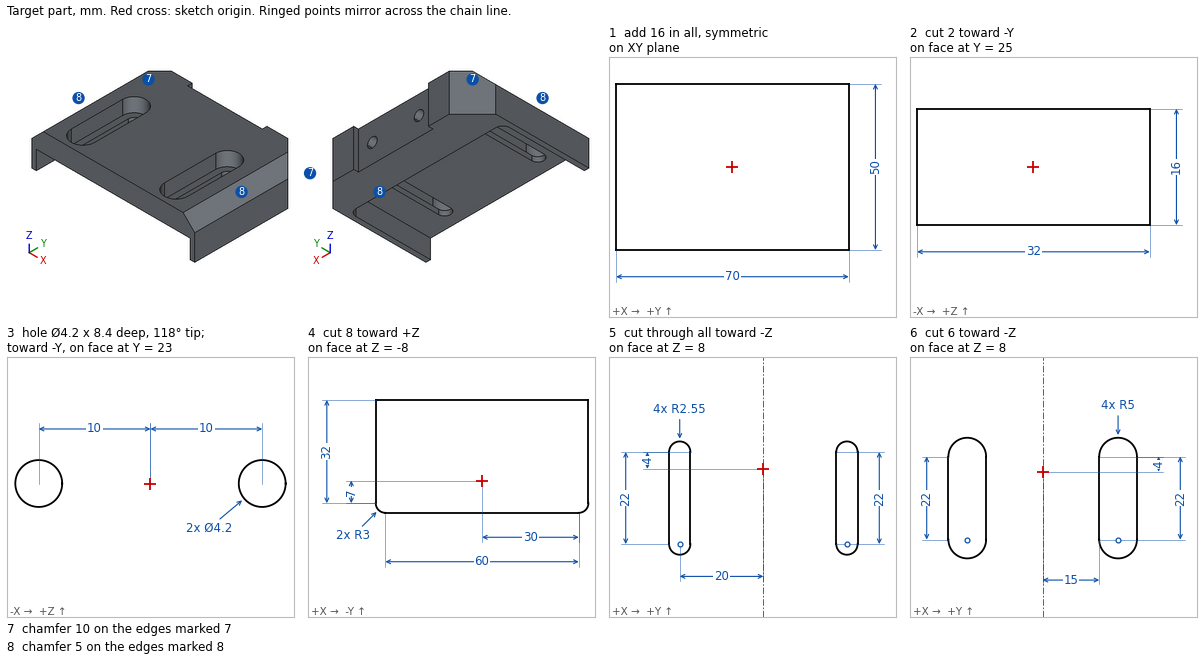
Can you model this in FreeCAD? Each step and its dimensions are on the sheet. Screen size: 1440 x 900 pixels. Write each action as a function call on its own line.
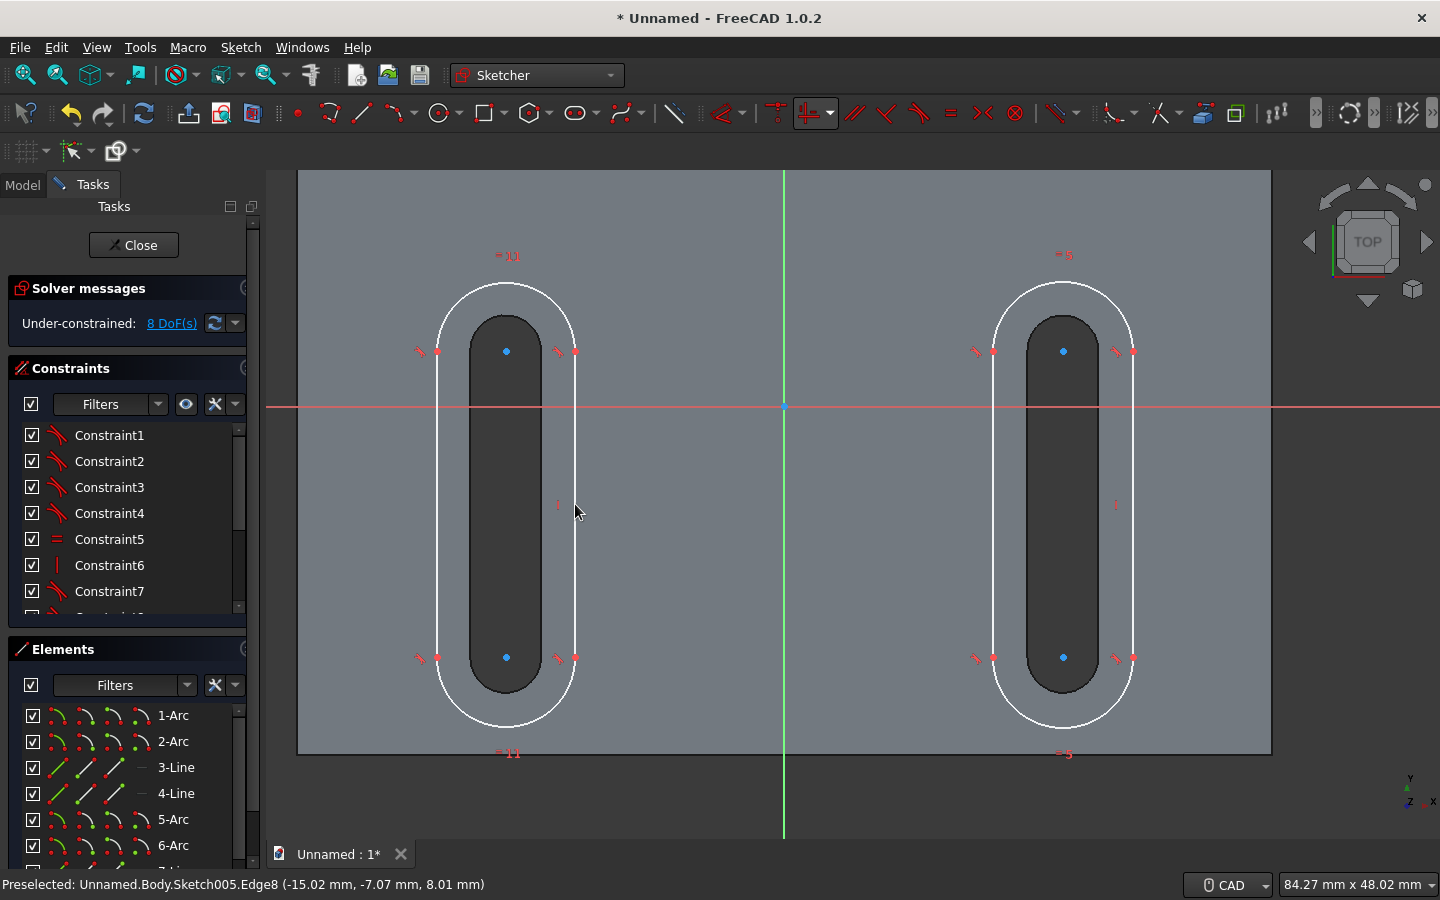
click(1022, 715)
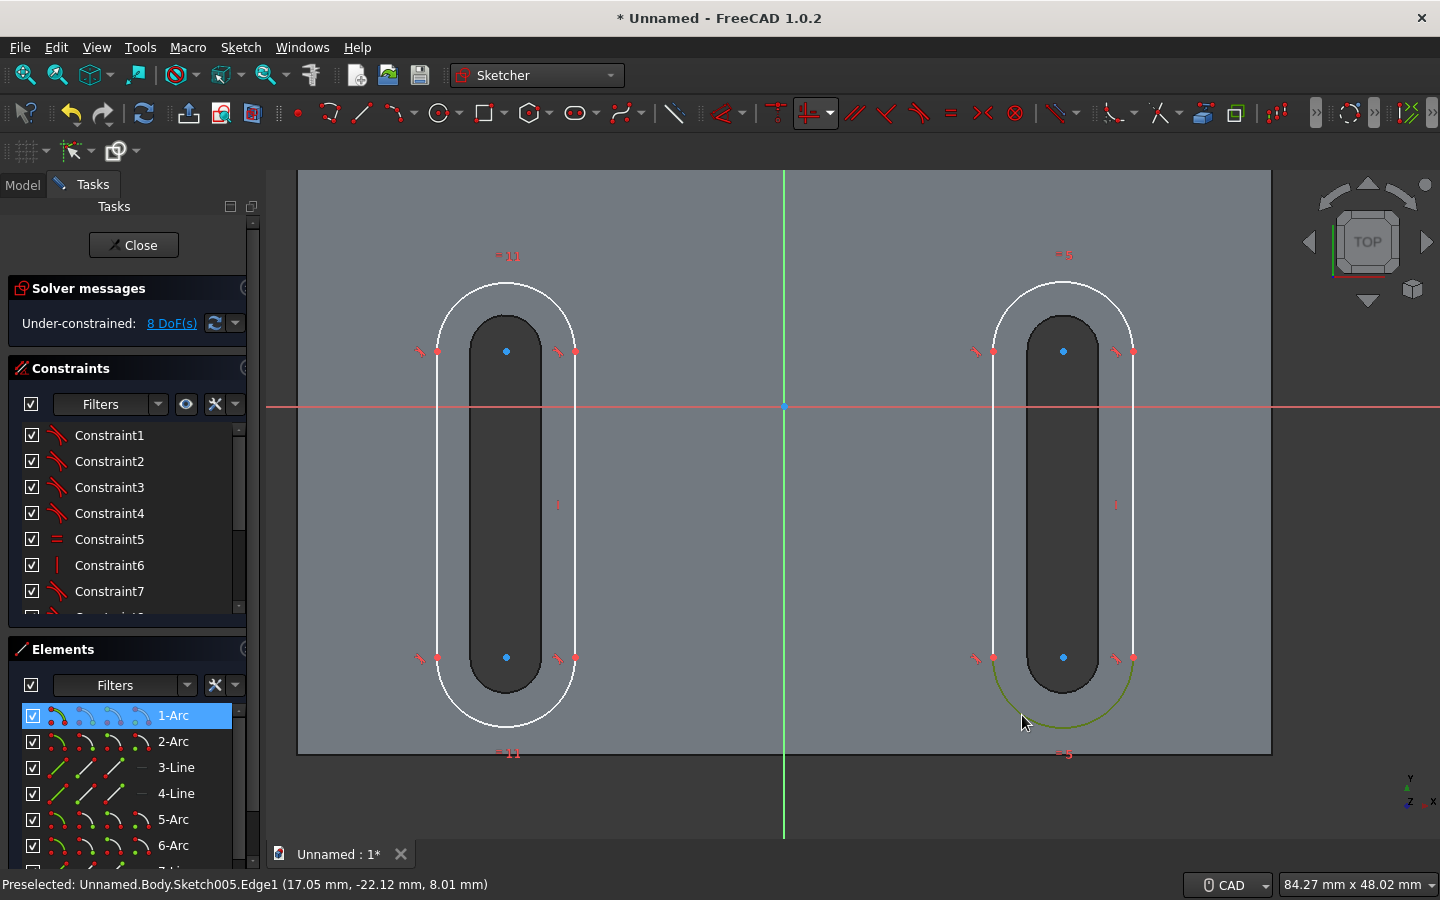
click(465, 714)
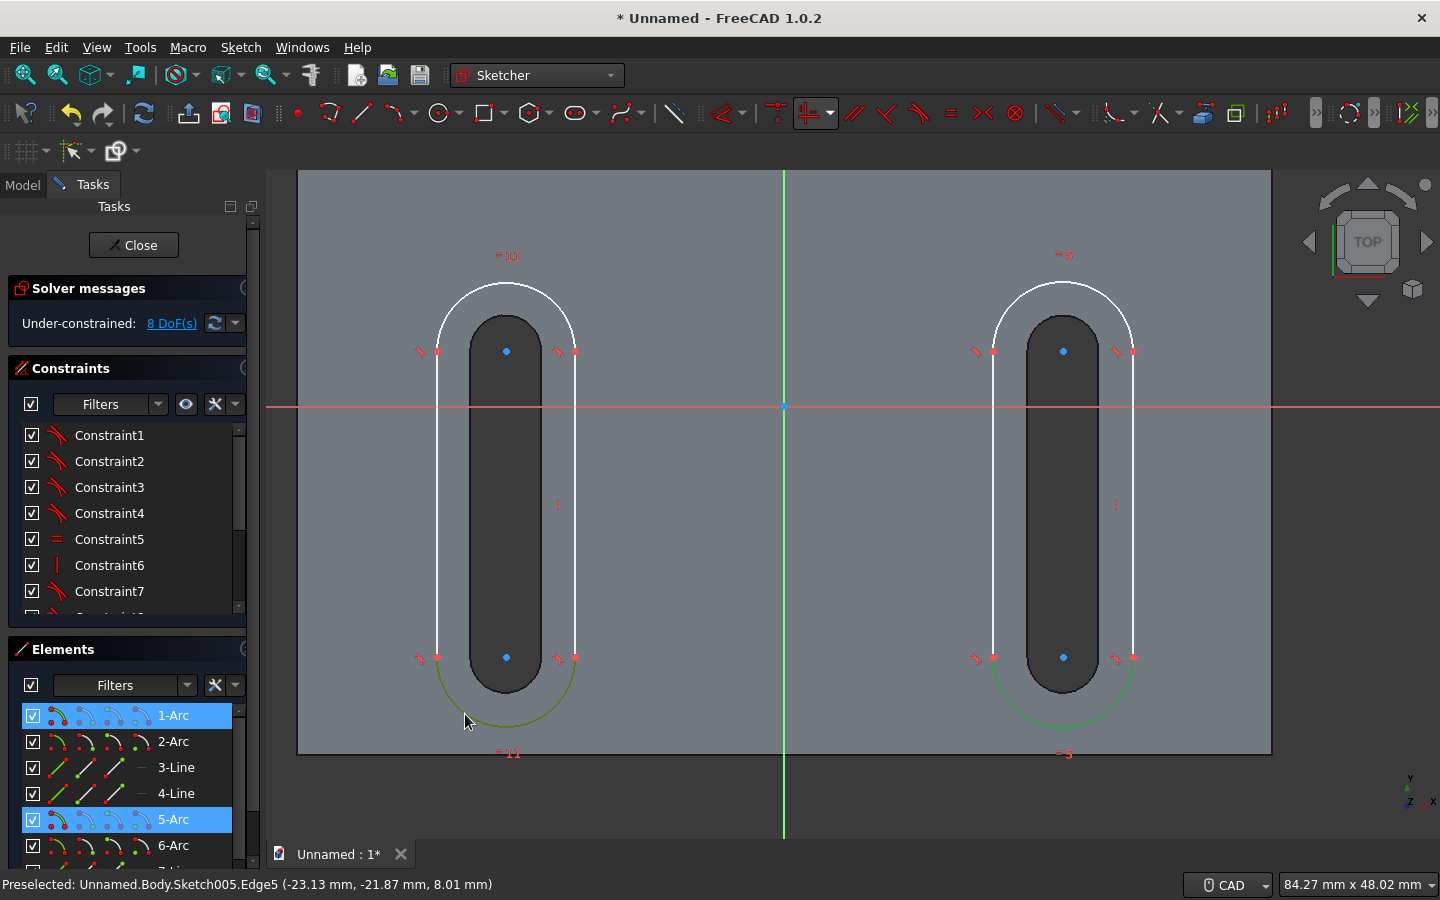
click(952, 114)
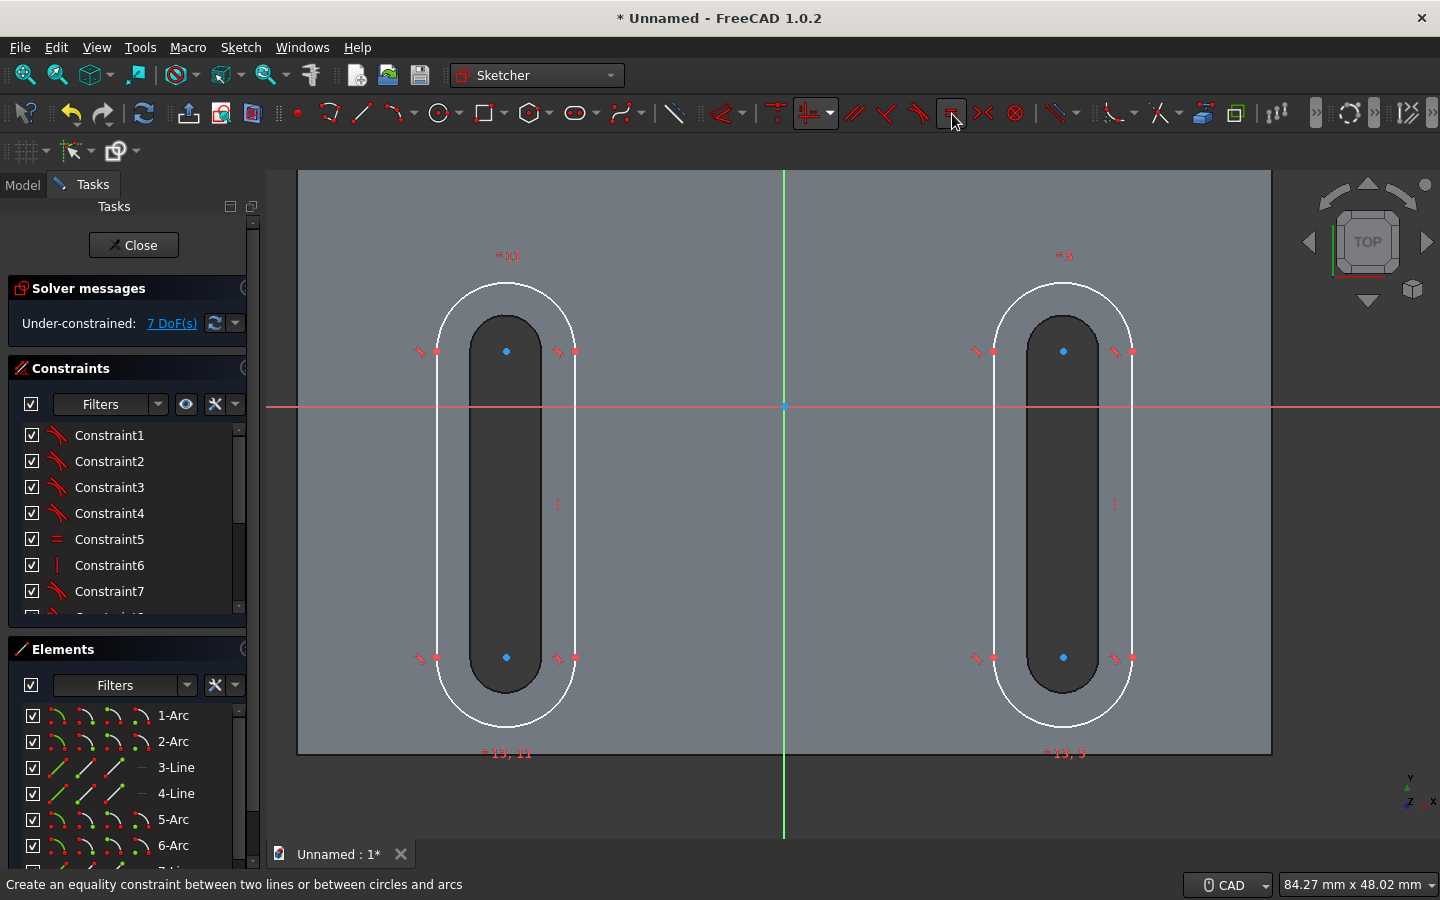
click(1063, 658)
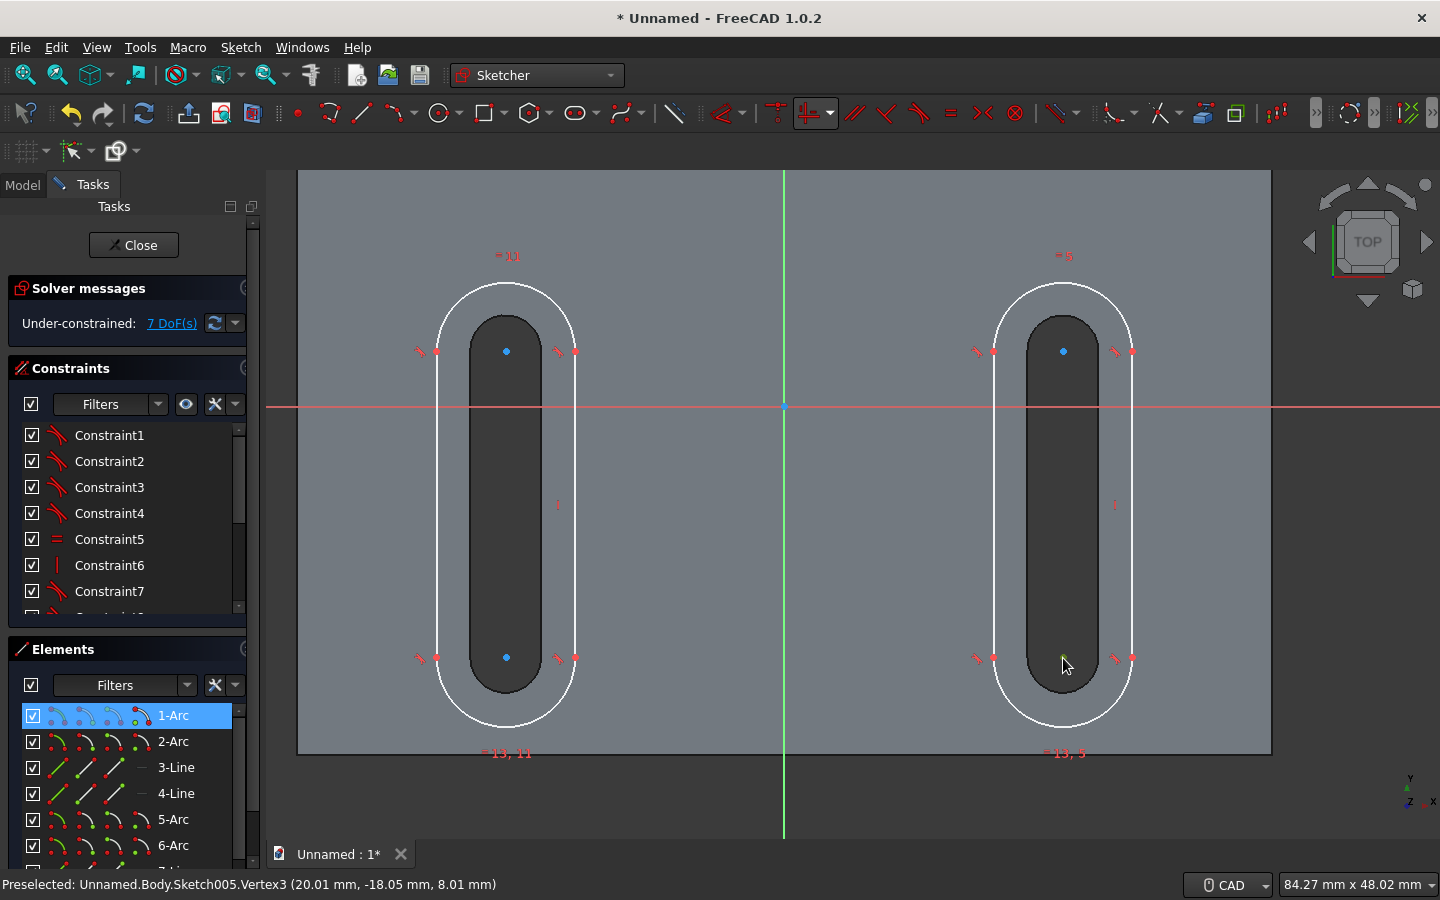
click(506, 658)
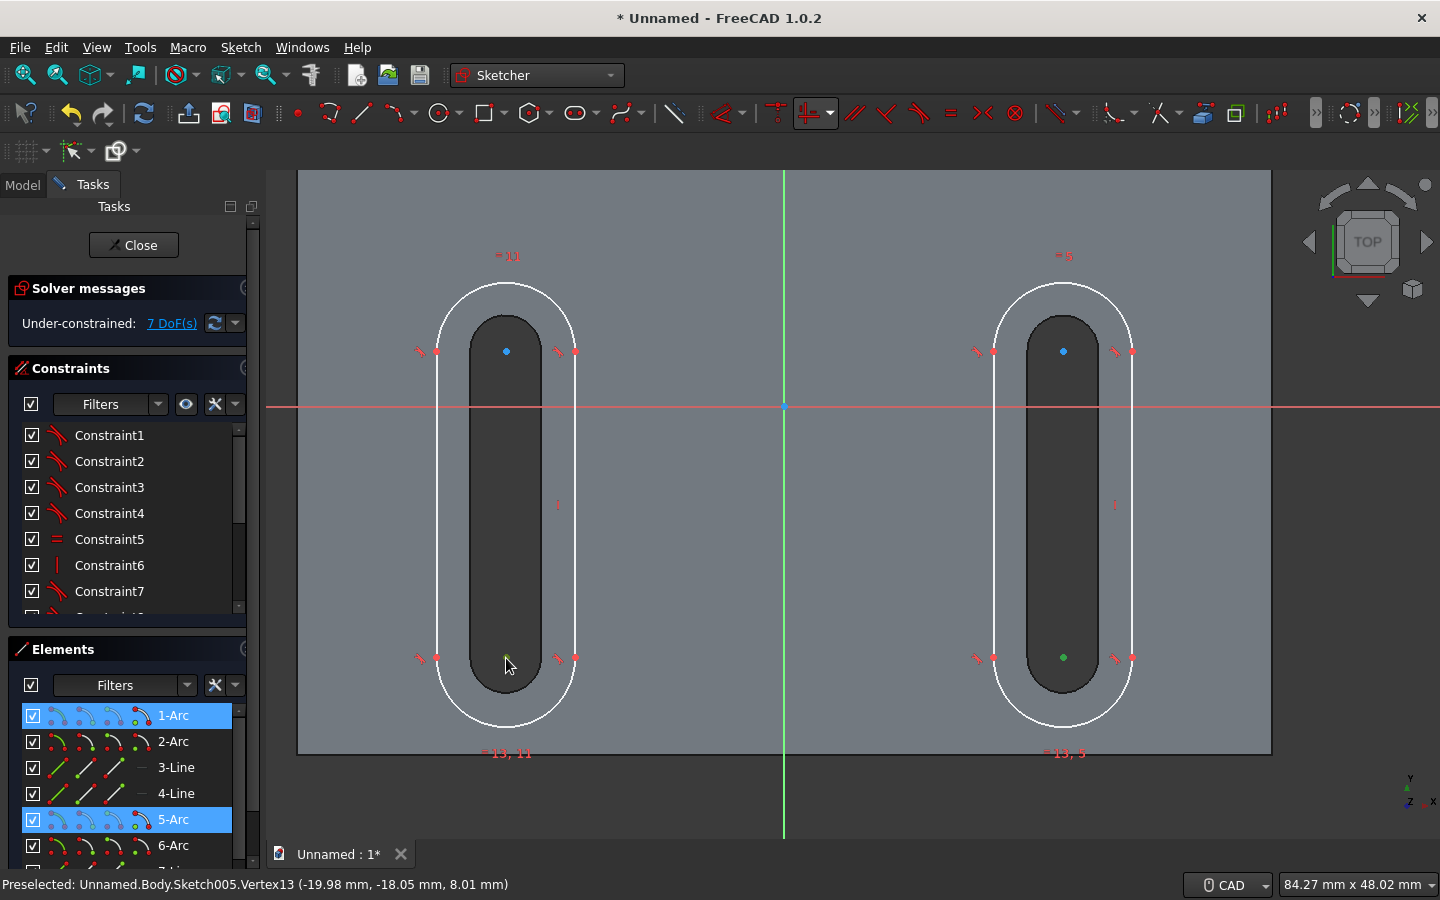
click(784, 767)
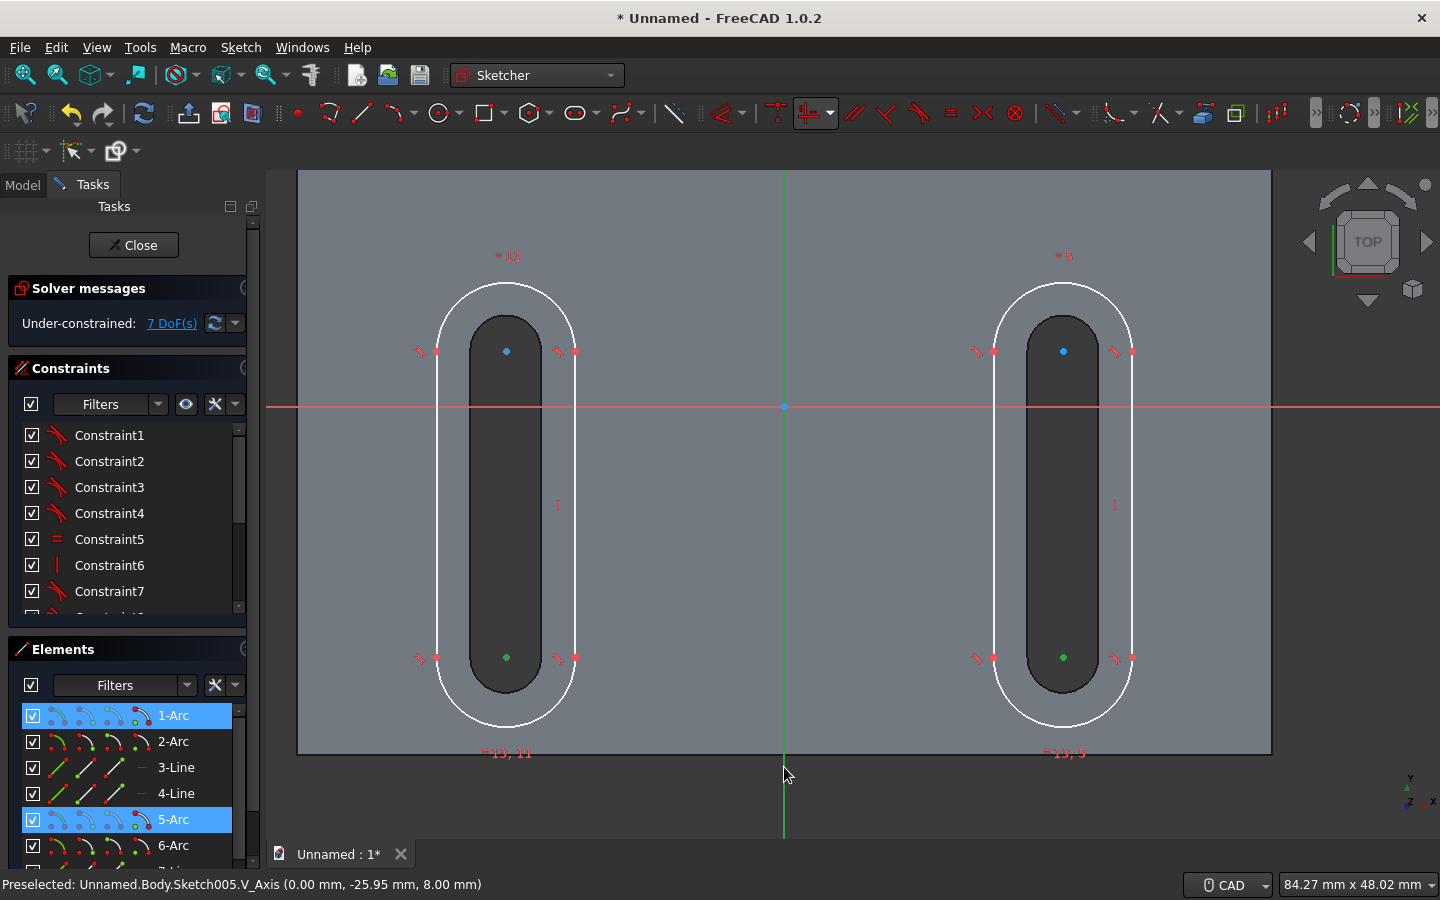
click(984, 114)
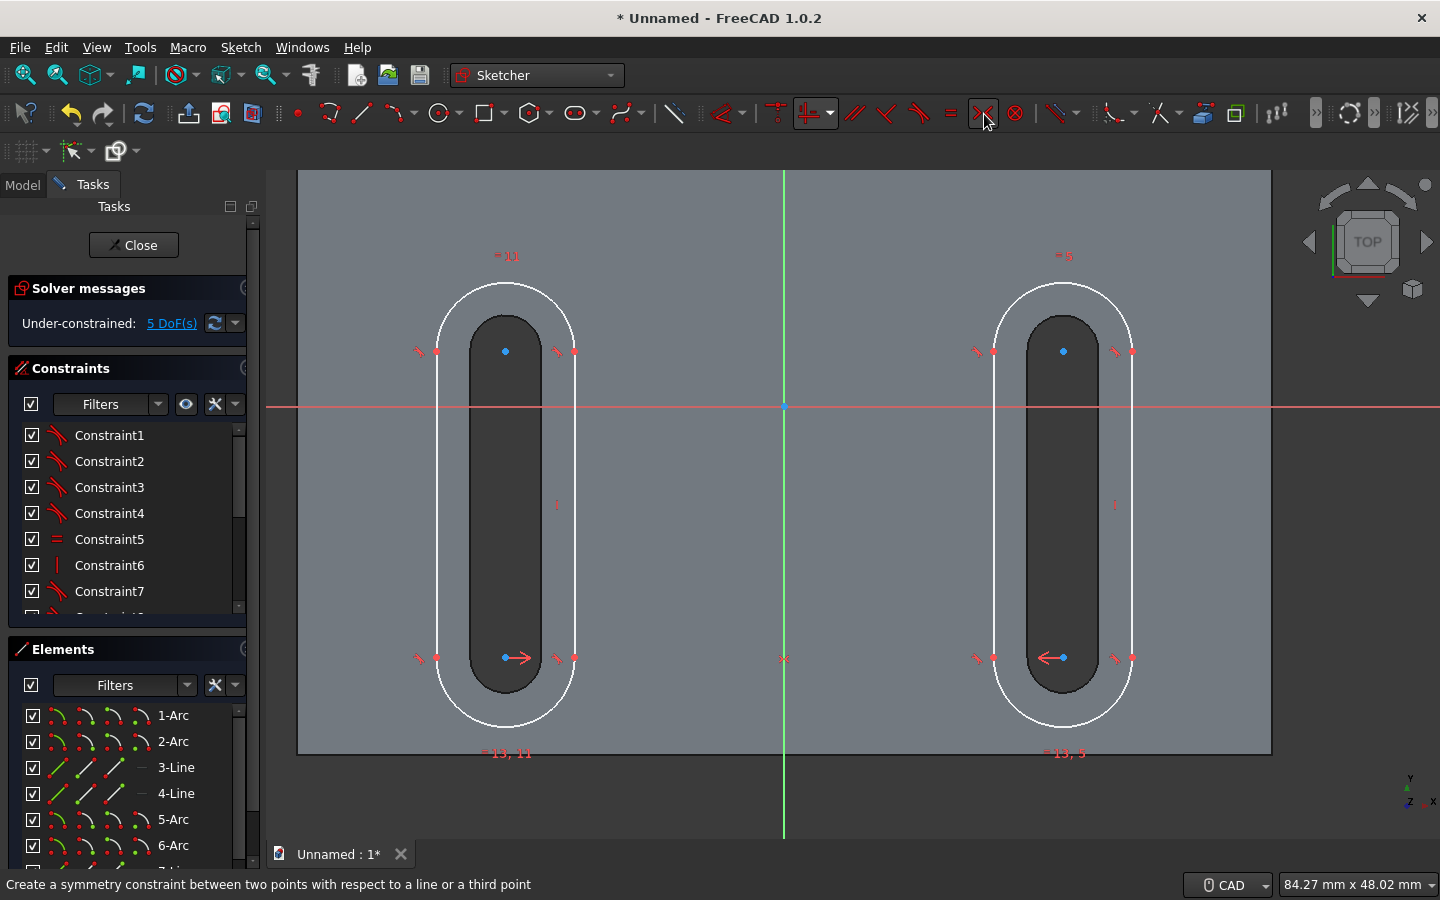
click(722, 114)